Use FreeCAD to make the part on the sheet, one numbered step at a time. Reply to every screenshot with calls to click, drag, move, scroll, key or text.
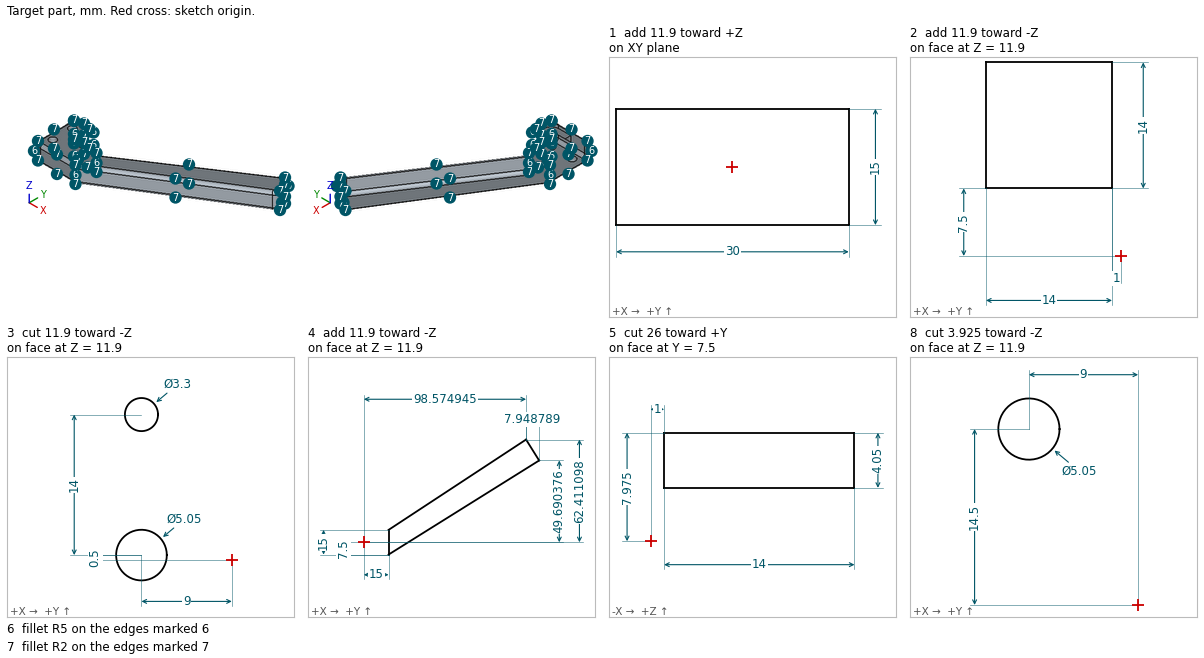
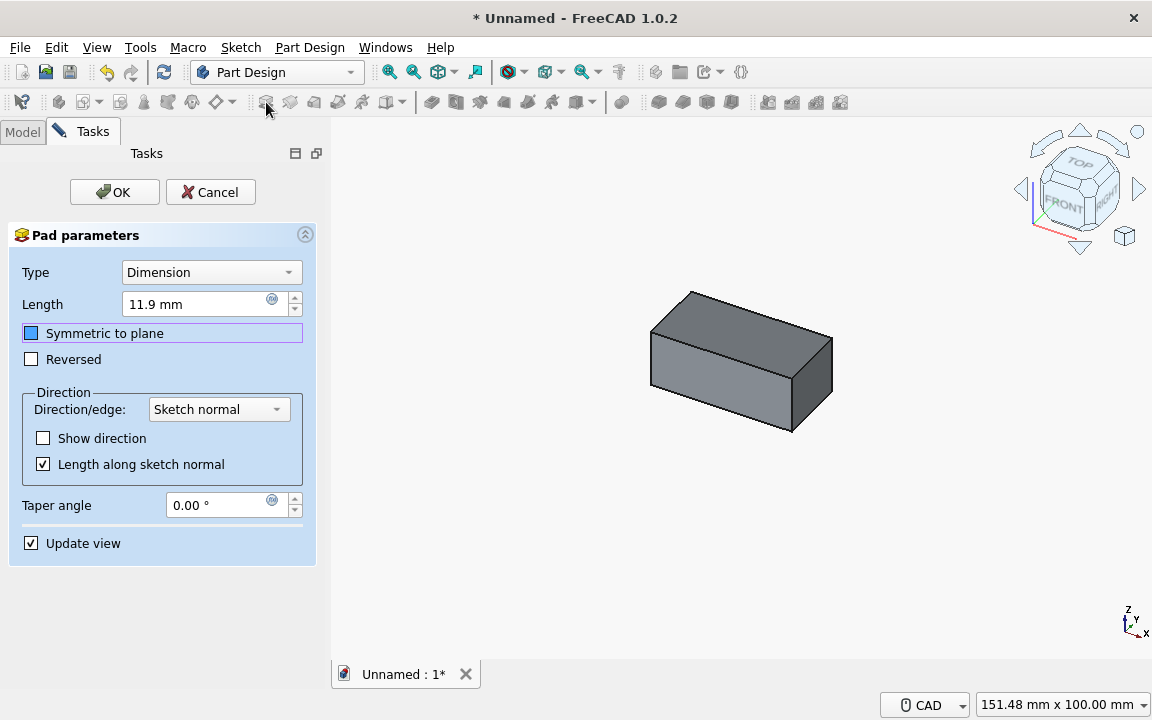
click(115, 192)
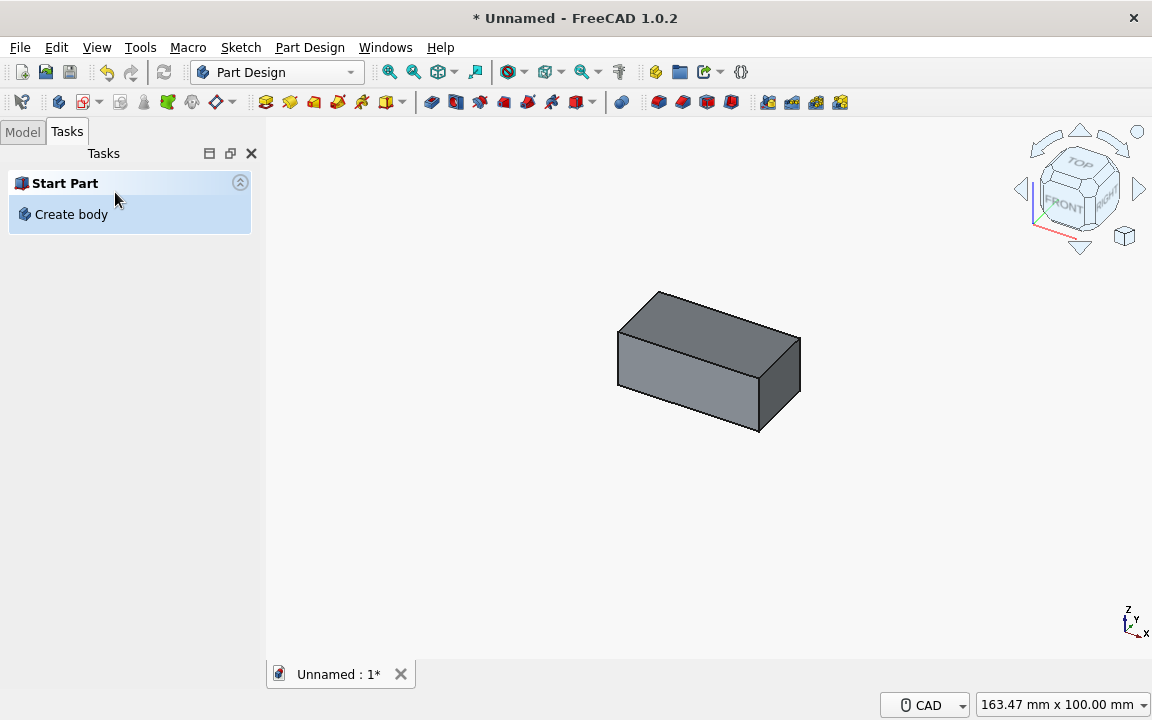
click(390, 72)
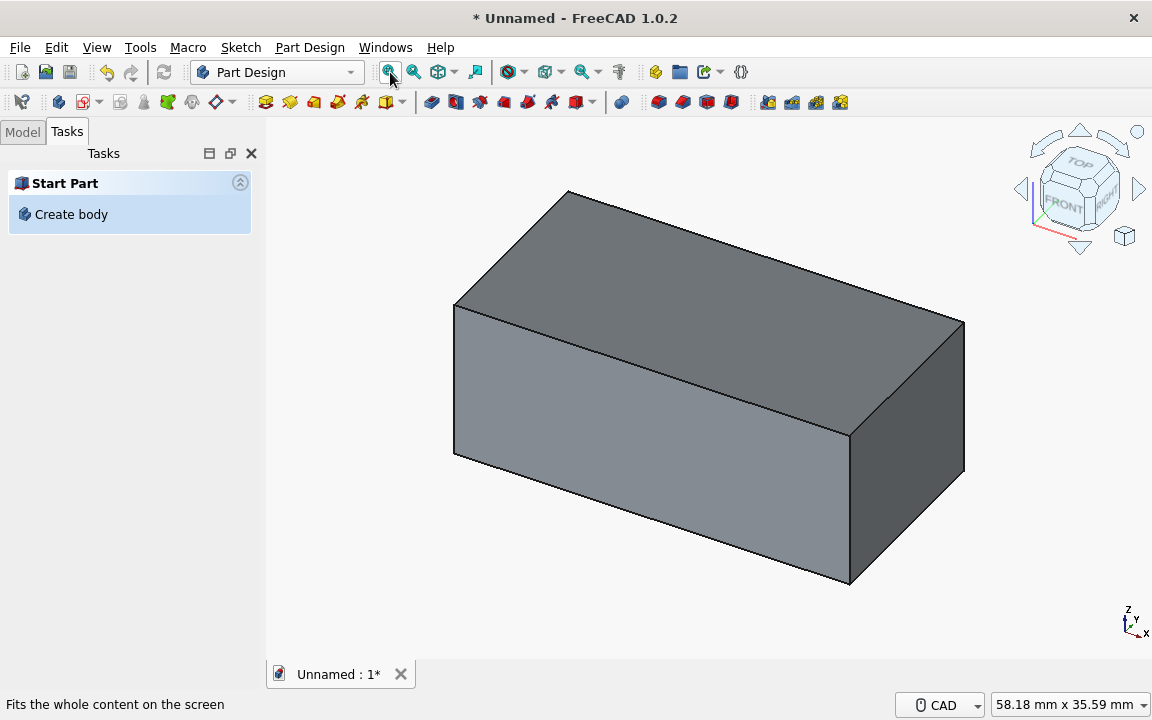
click(766, 331)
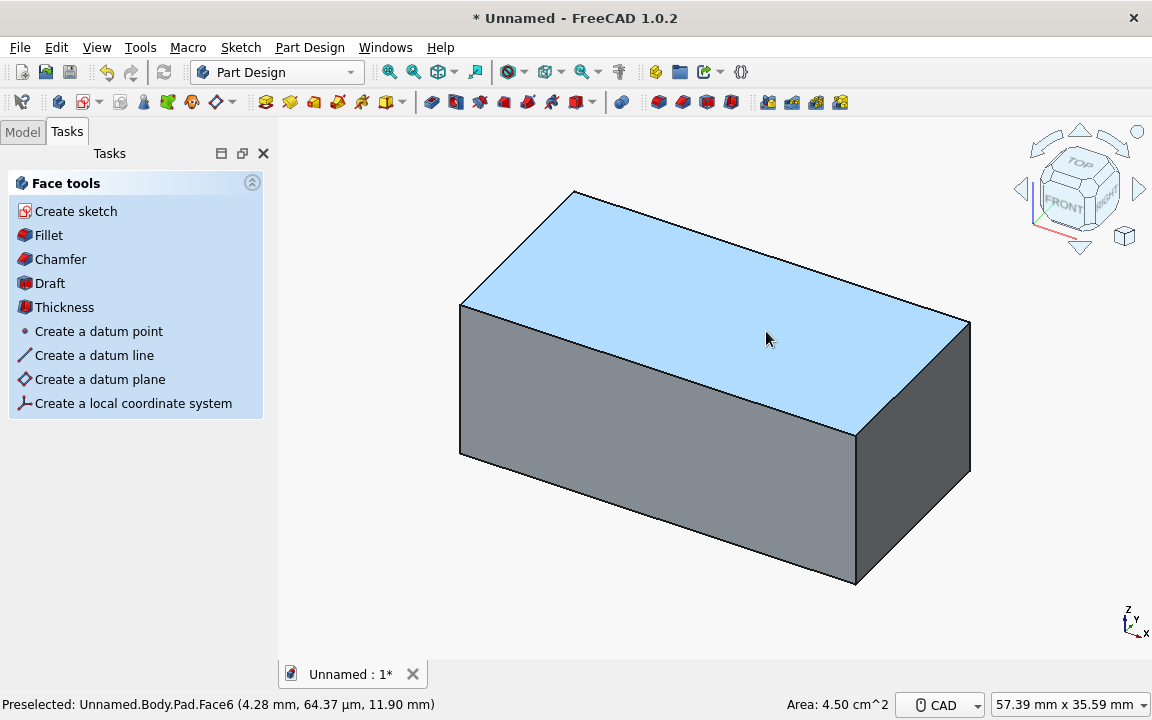
click(84, 102)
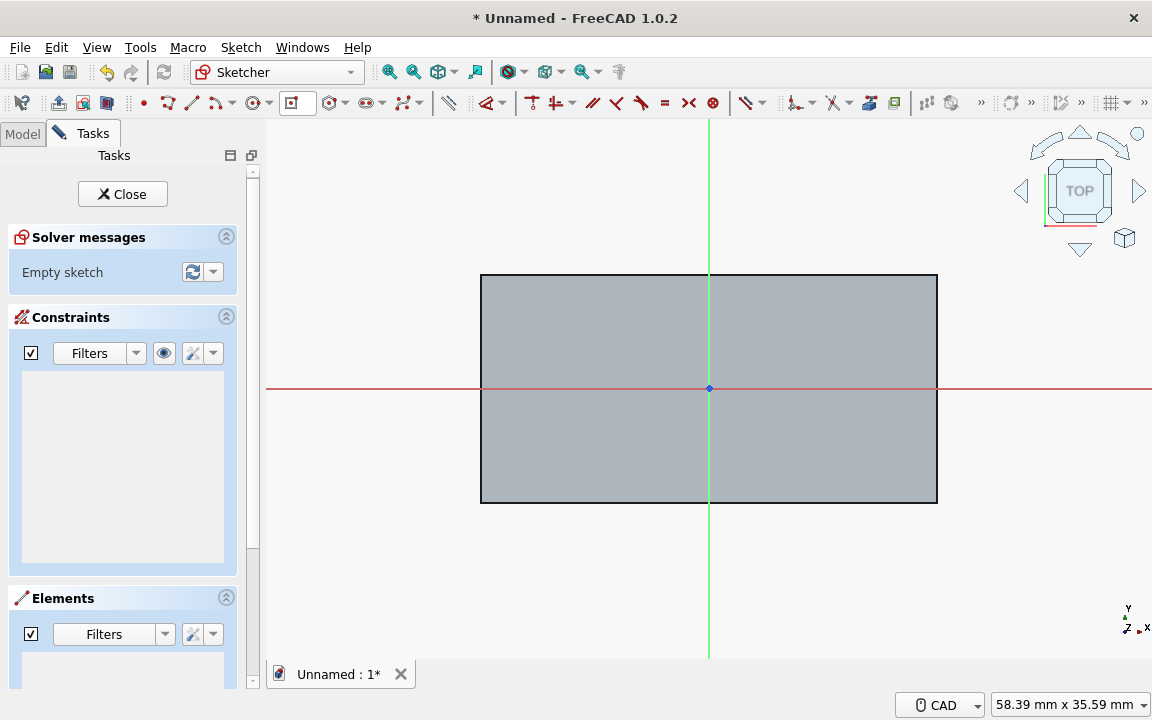
scroll(733, 631, down, 2)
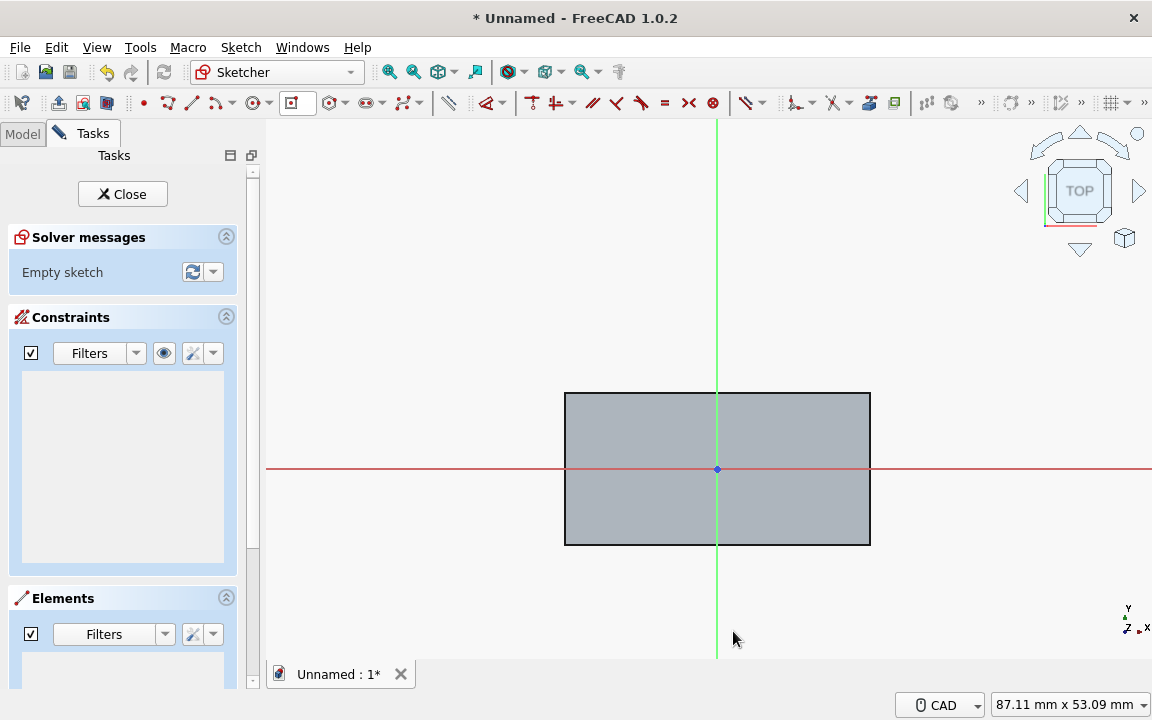
scroll(641, 300, up, 2)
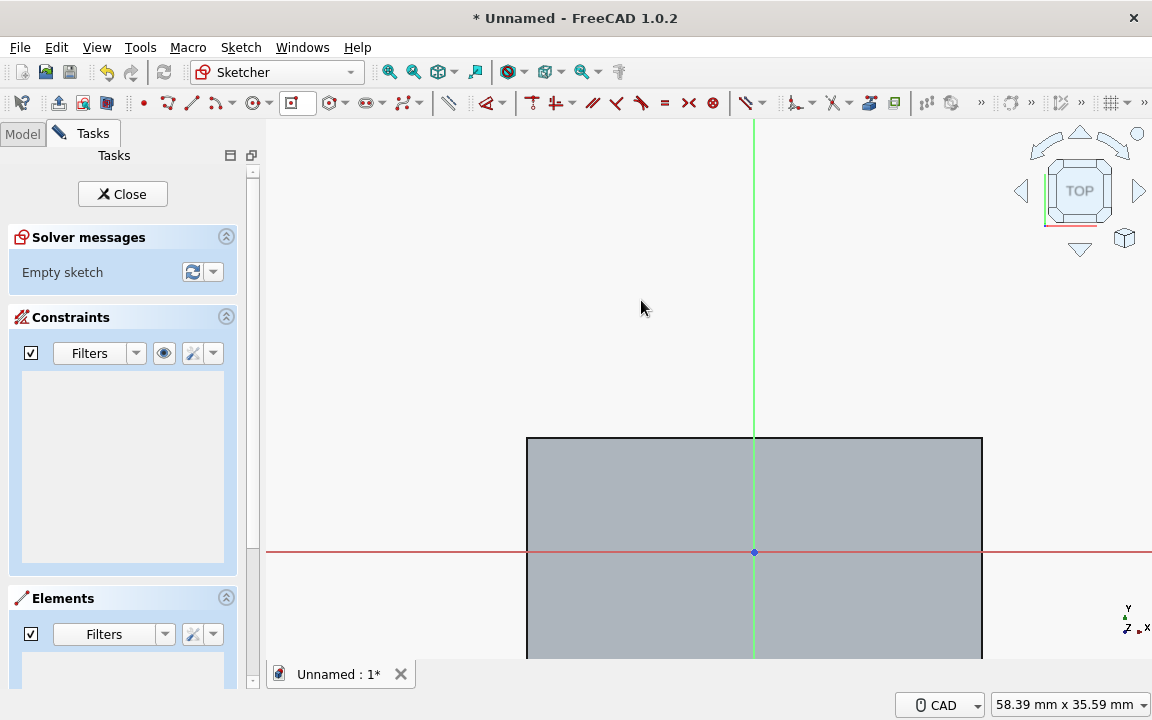
key(g)
key(r)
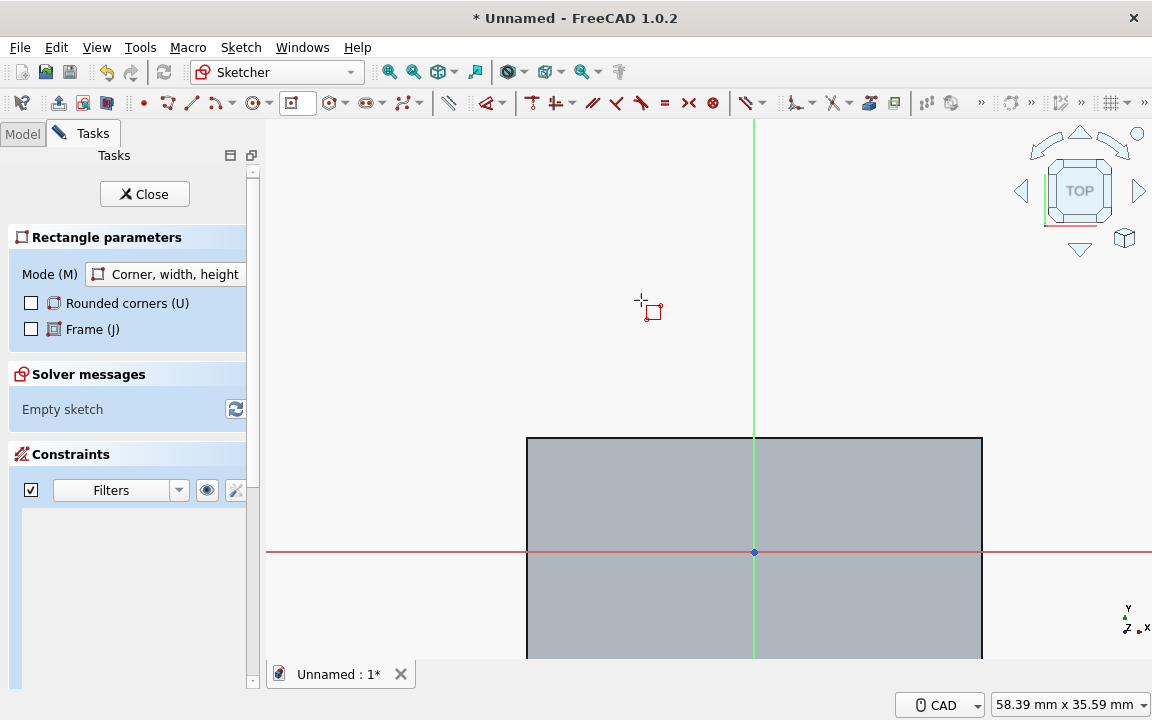
click(527, 226)
move(739, 438)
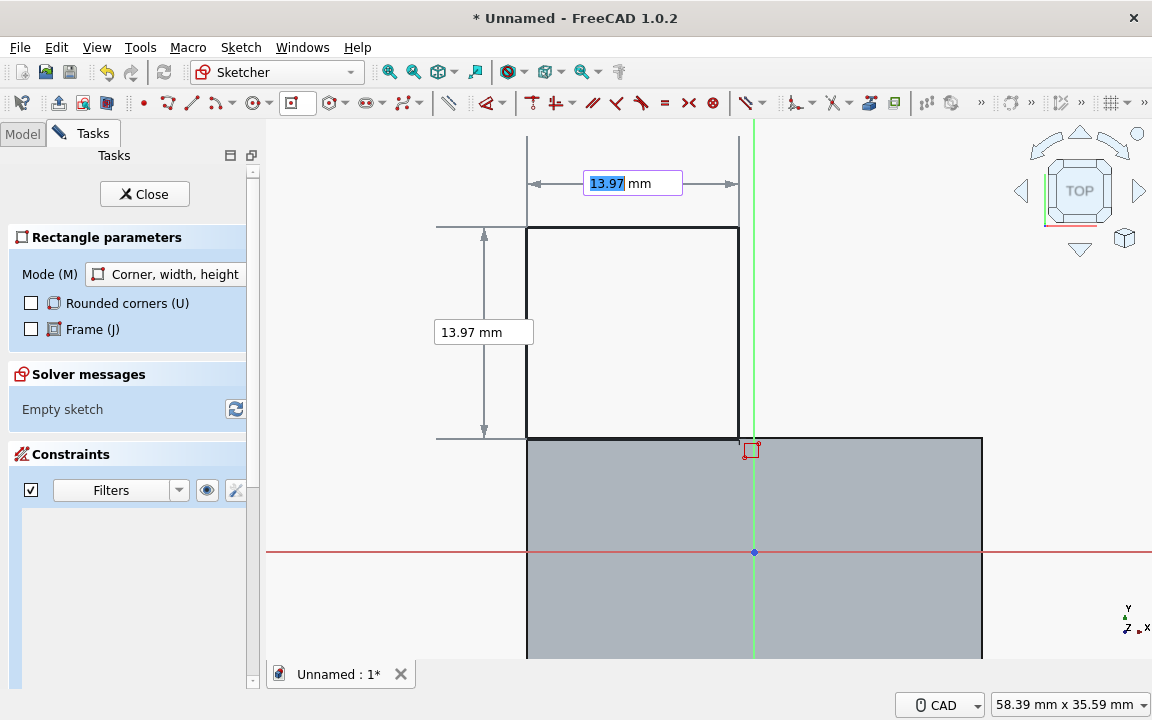
text(14)
key(Tab)
text(14)
key(Return)
key(Escape)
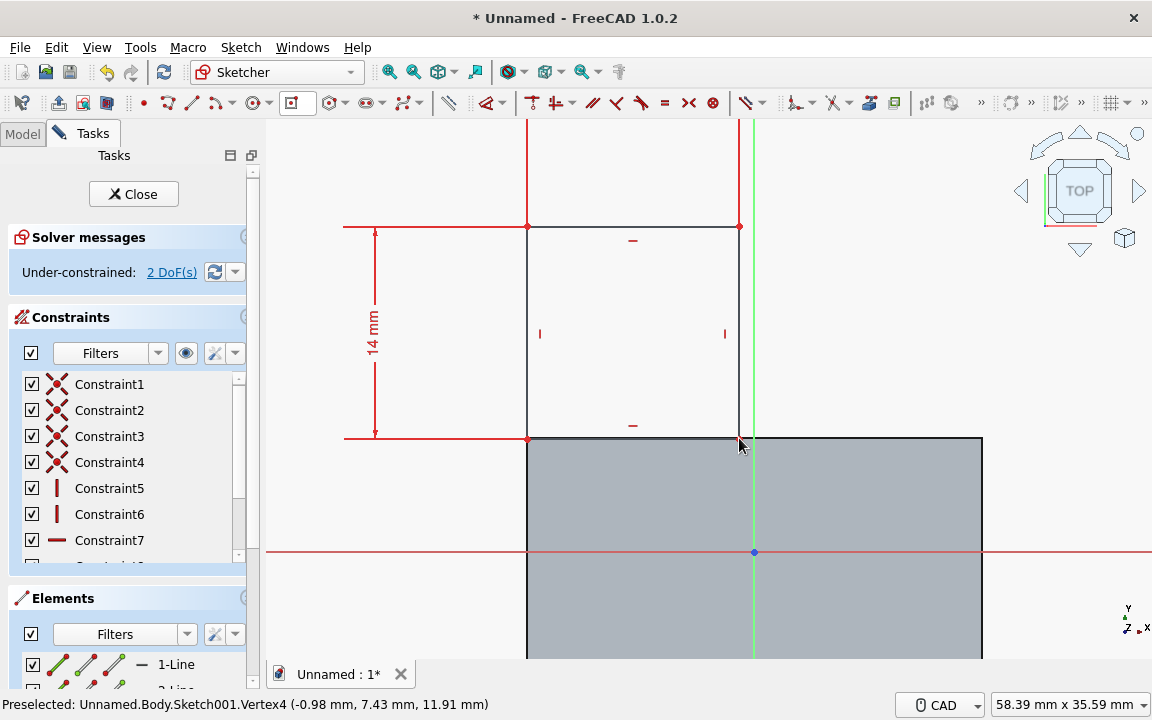
click(486, 104)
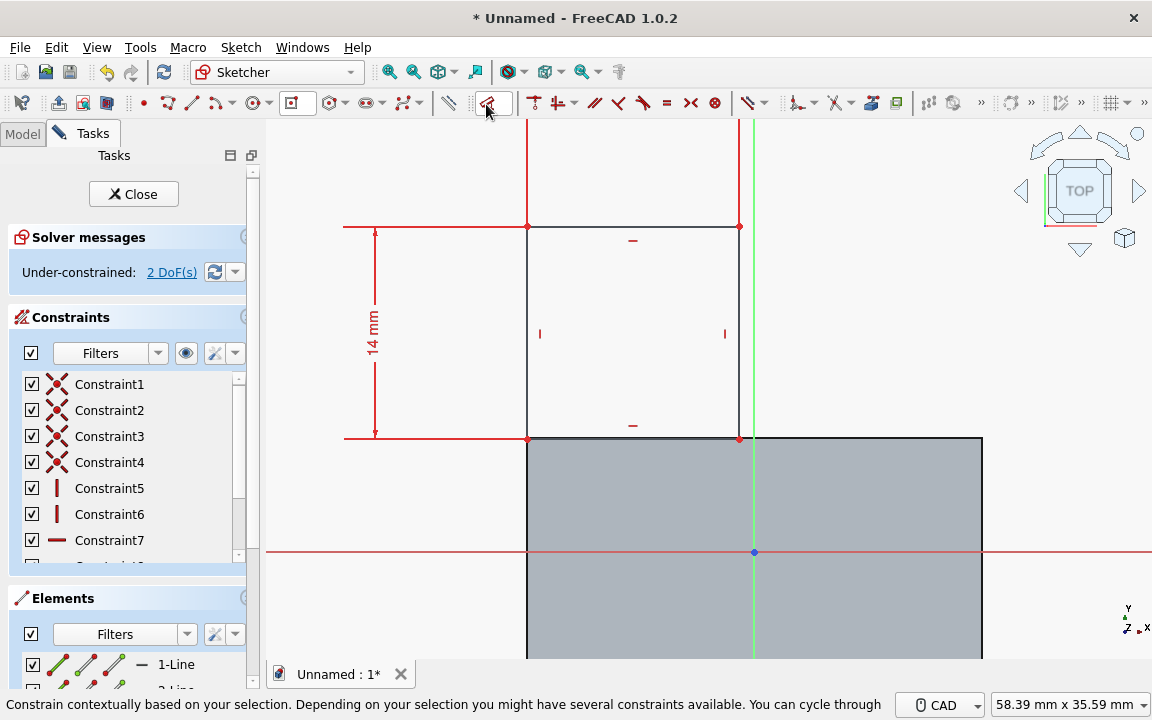
scroll(739, 439, up, 5)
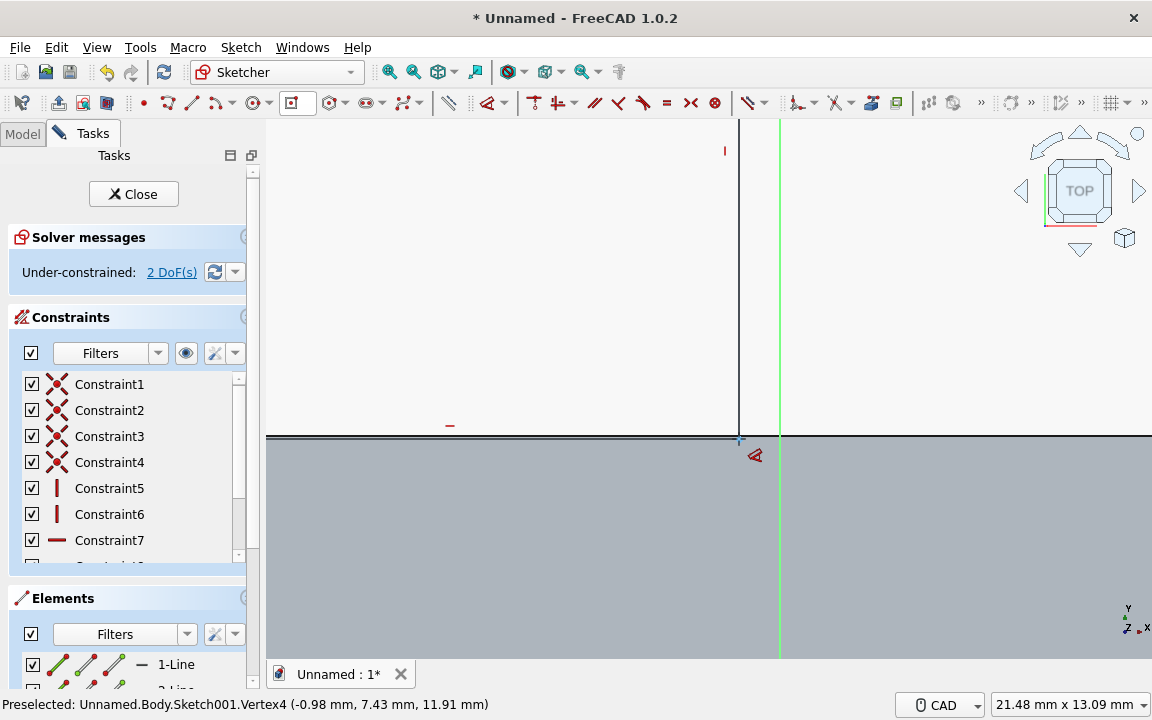
click(739, 439)
click(759, 405)